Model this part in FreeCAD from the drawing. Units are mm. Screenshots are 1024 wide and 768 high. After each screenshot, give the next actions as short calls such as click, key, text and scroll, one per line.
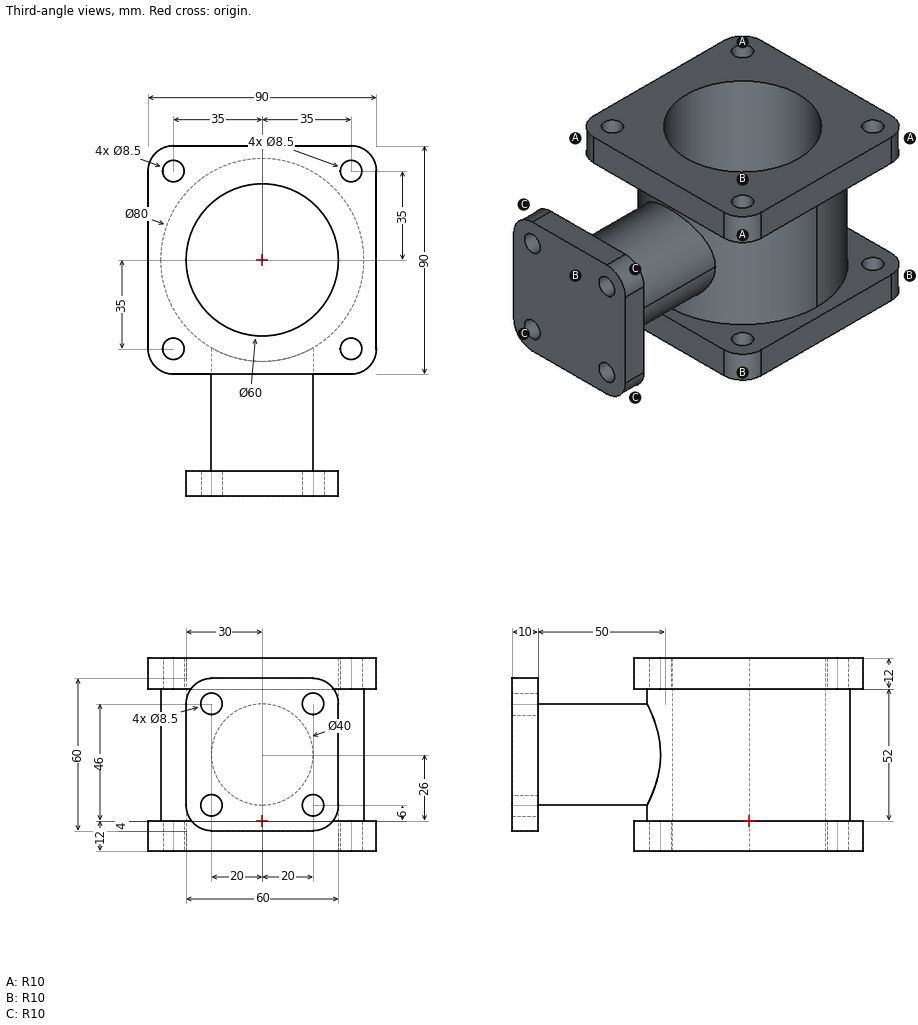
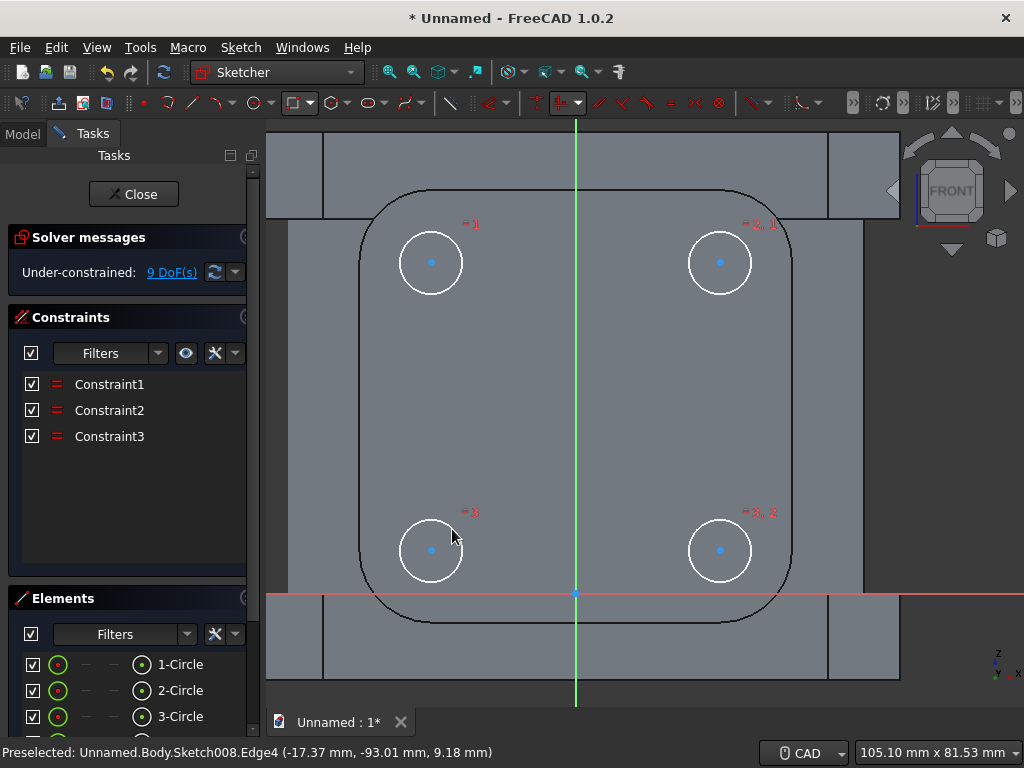
click(431, 263)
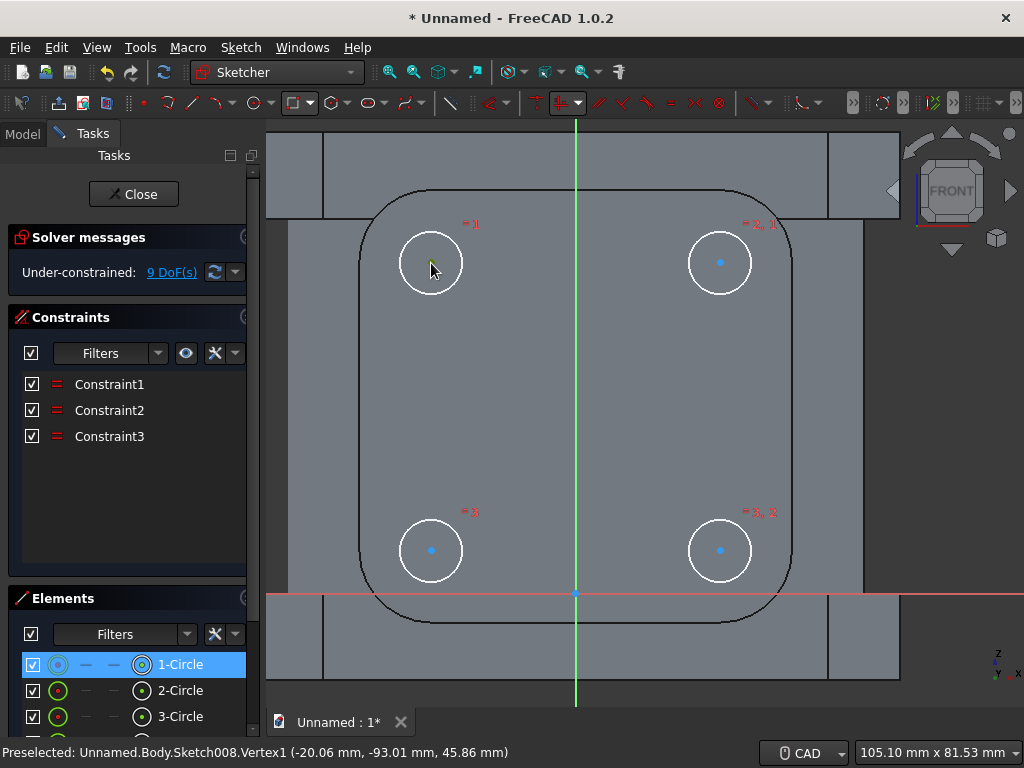
click(720, 263)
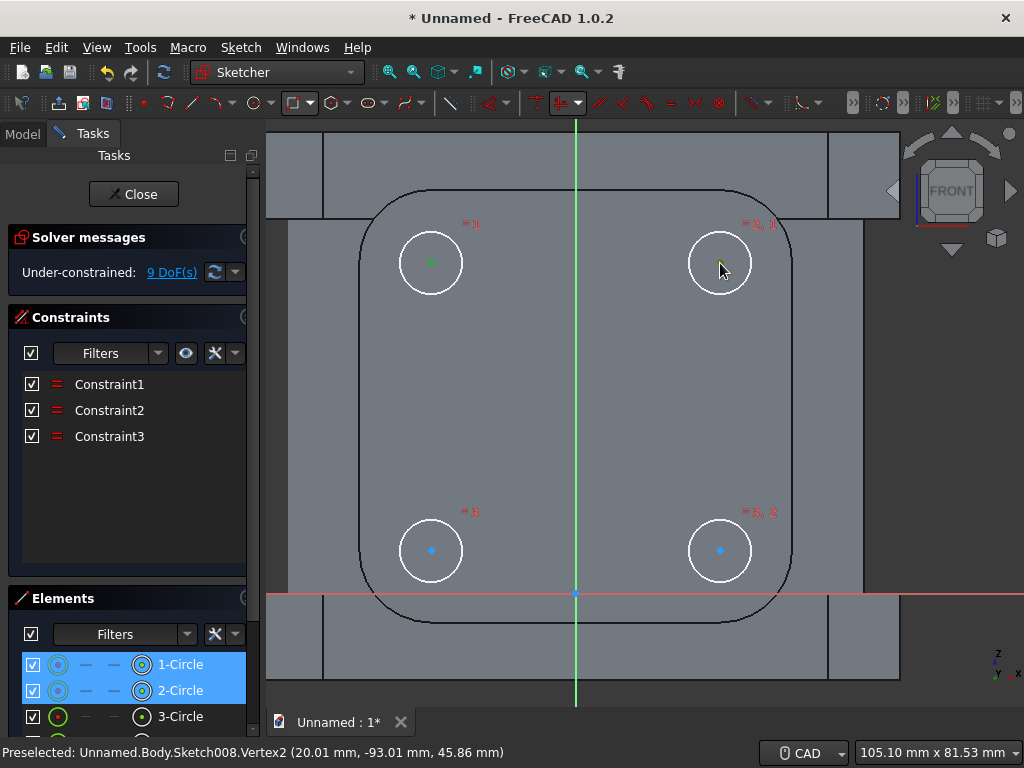
key(h)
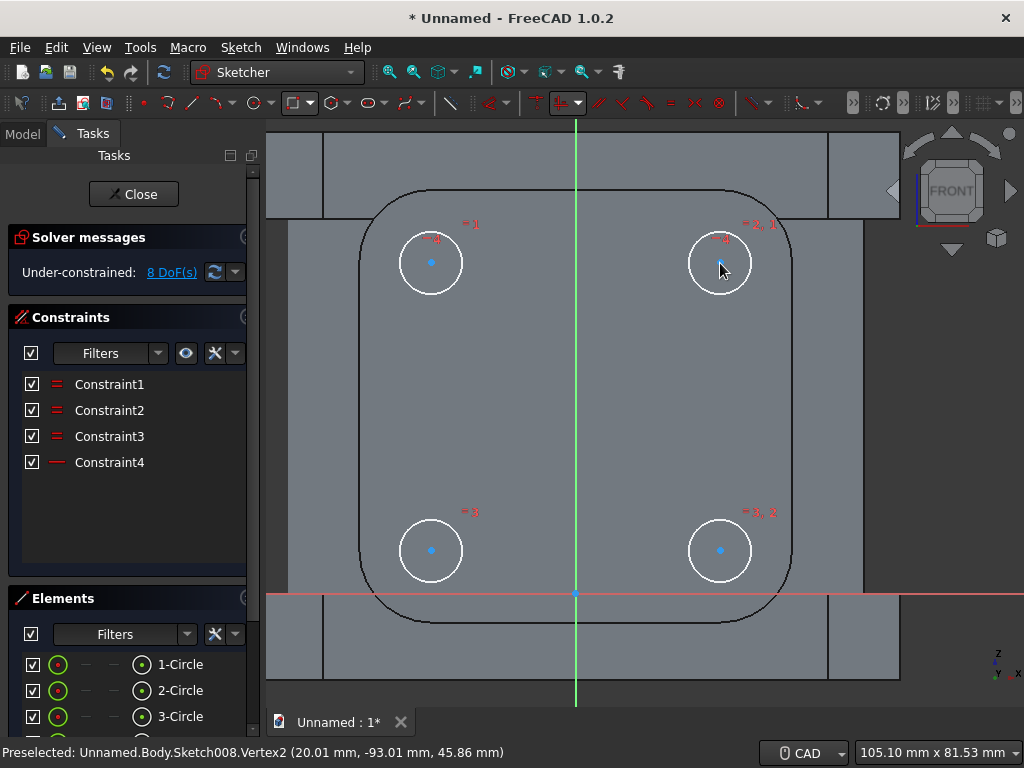
click(720, 263)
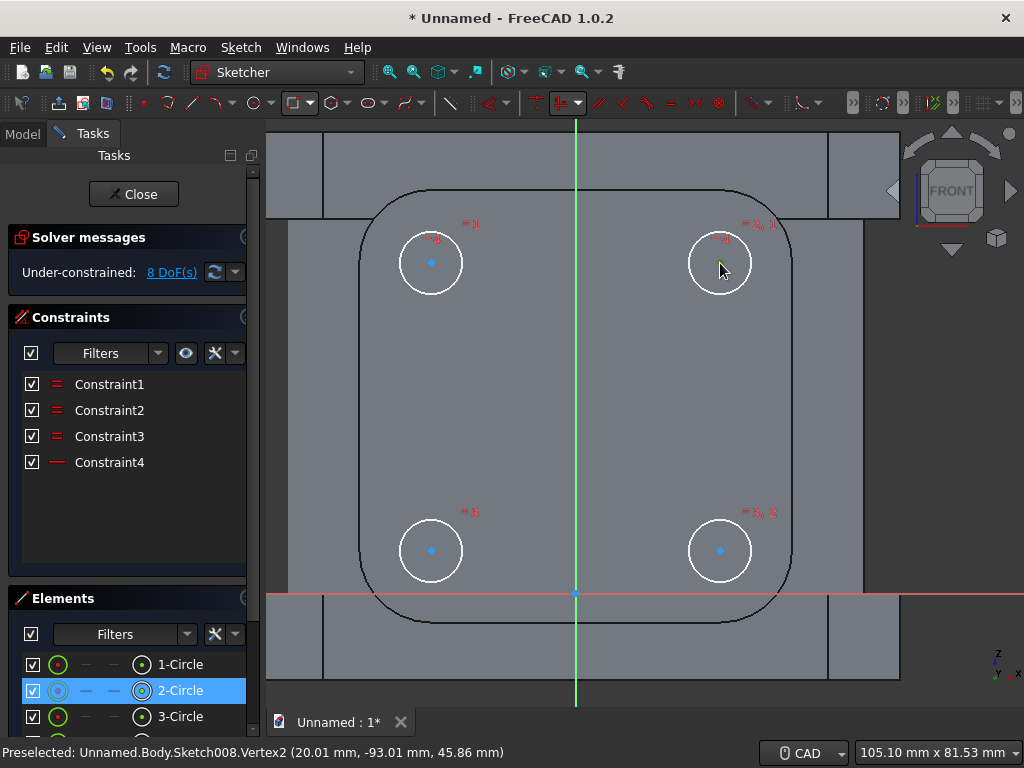
click(720, 551)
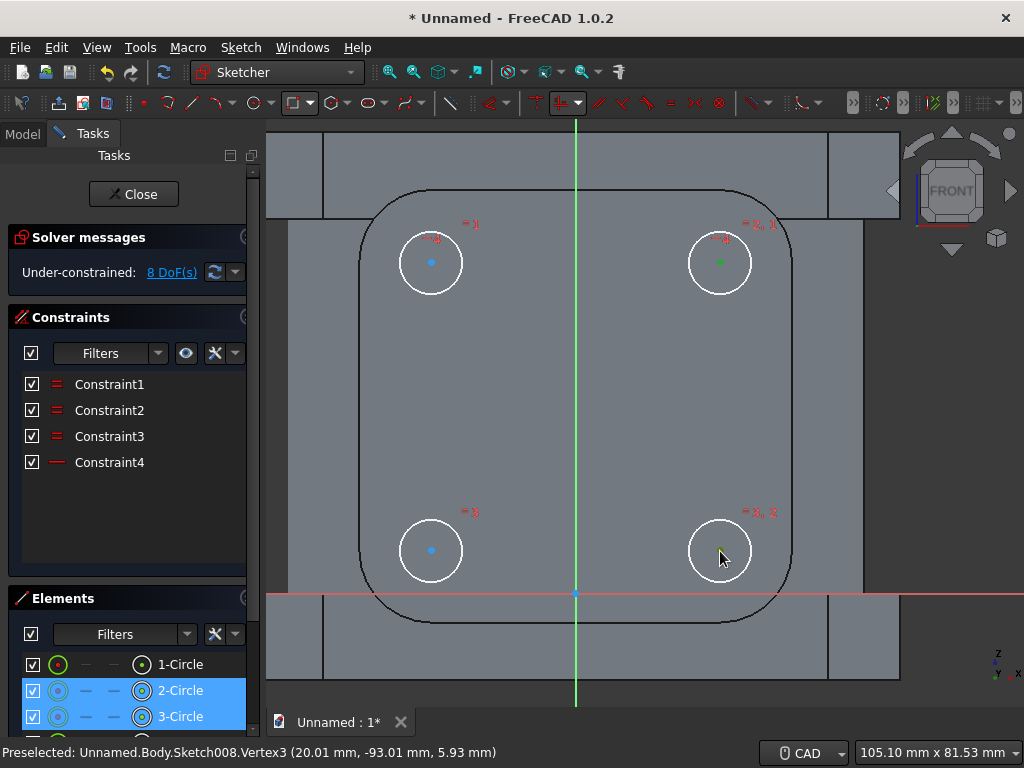
click(580, 104)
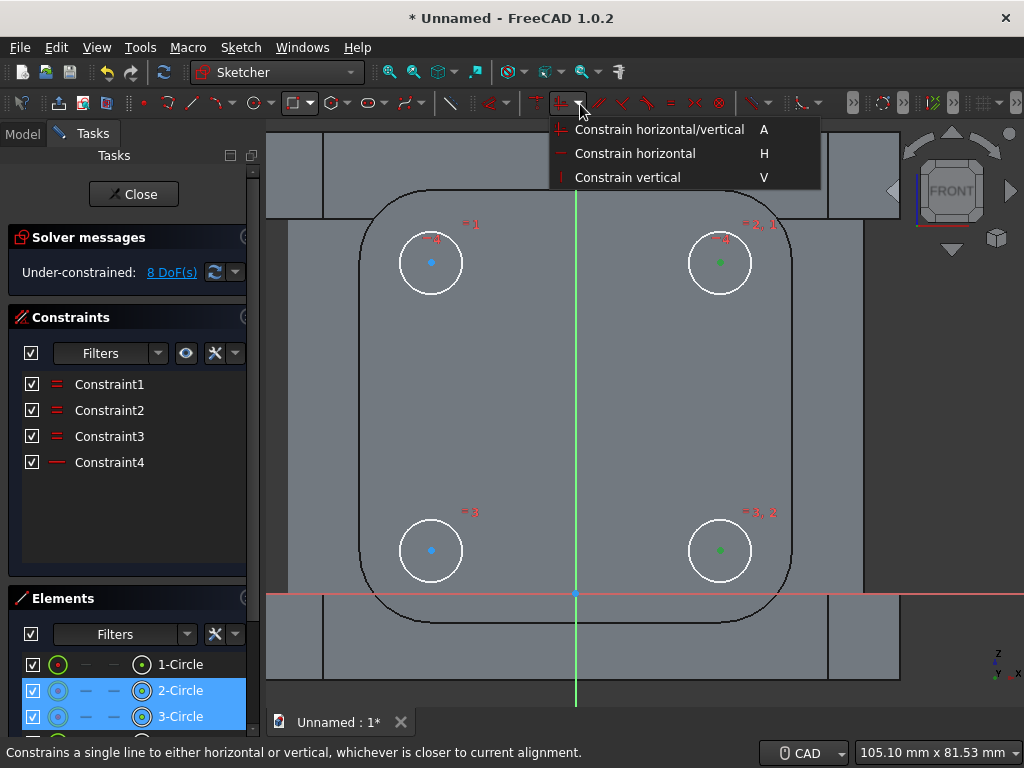
click(685, 177)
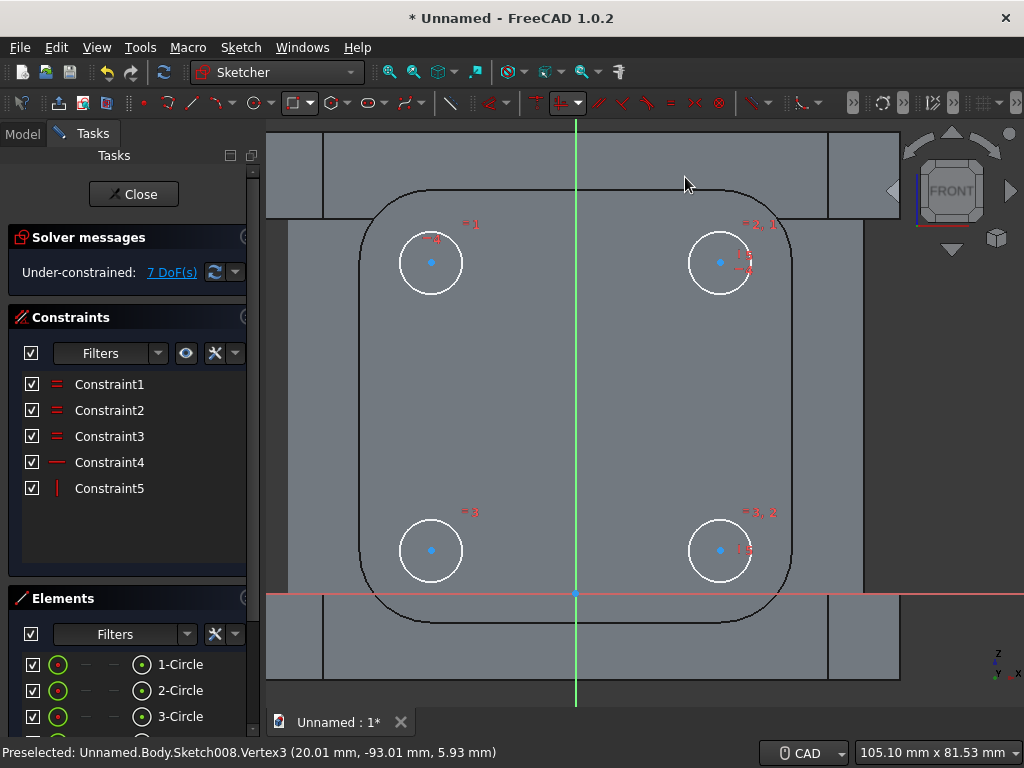
click(431, 263)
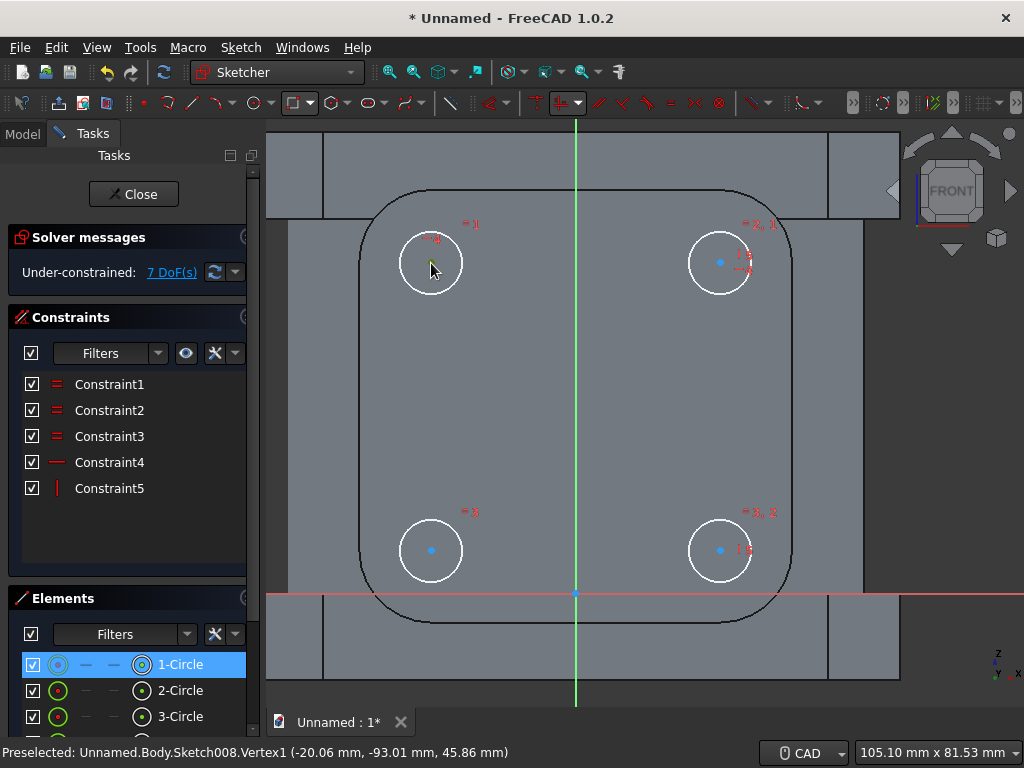
click(431, 551)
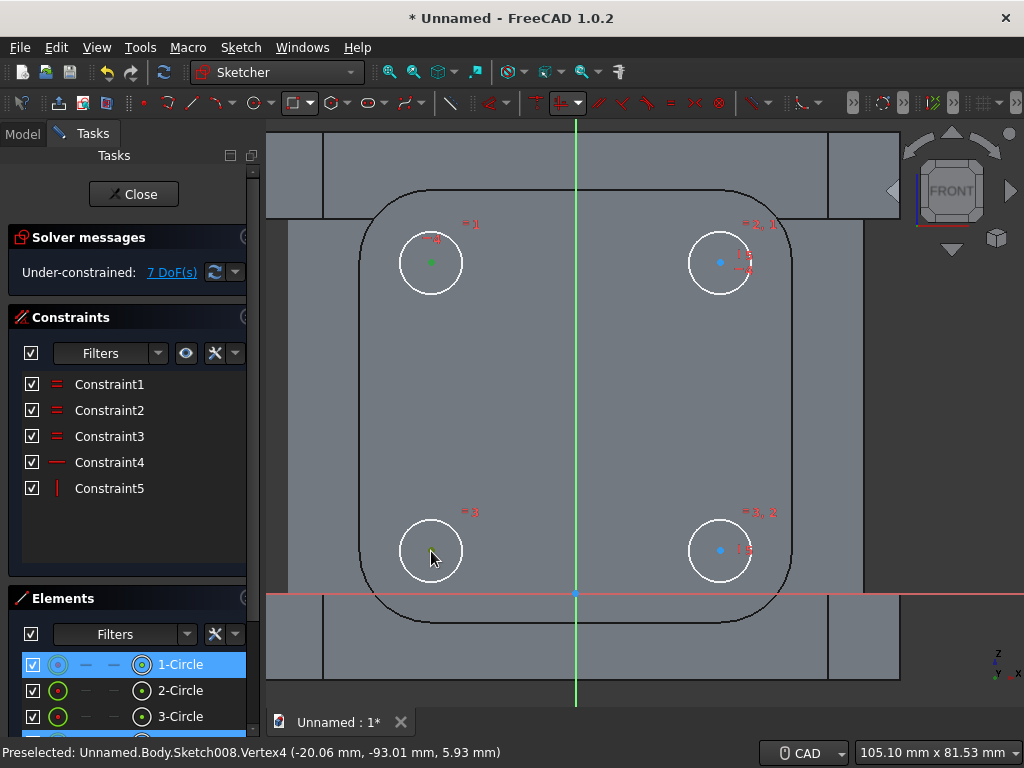
click(580, 104)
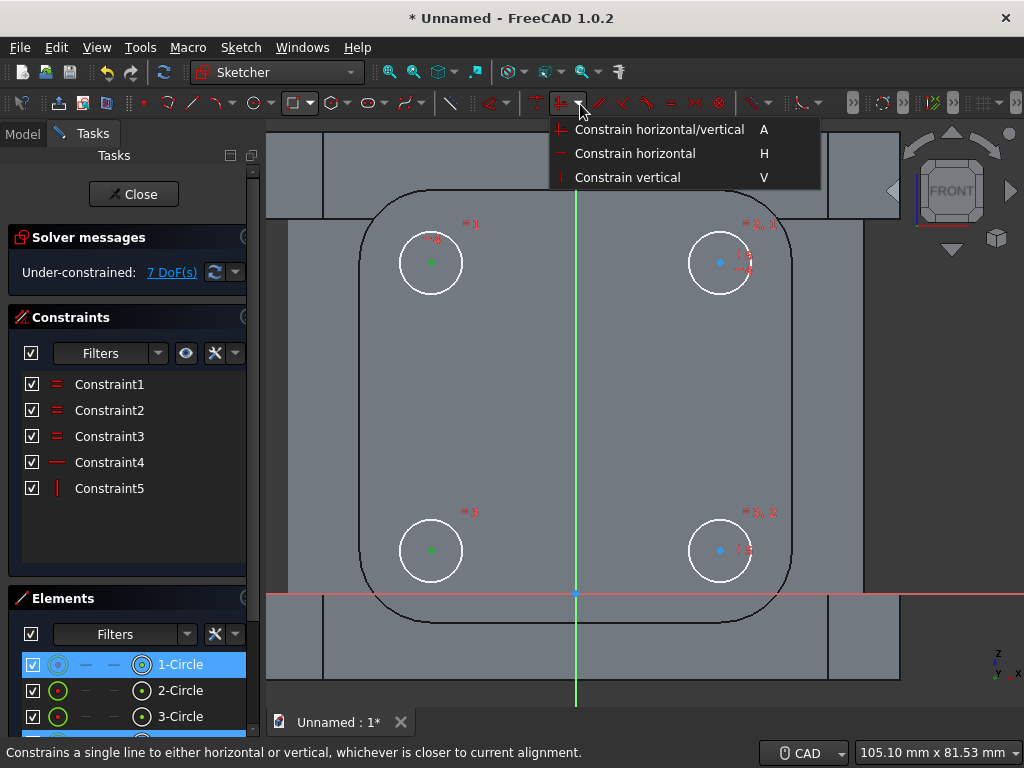
click(685, 177)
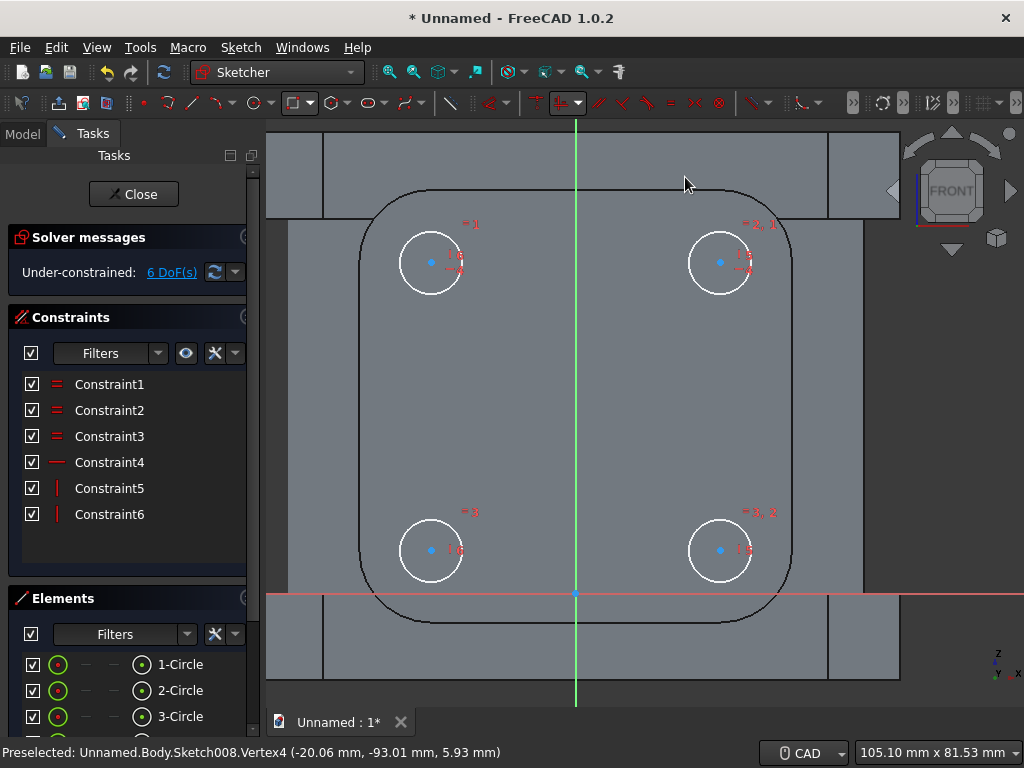
click(720, 551)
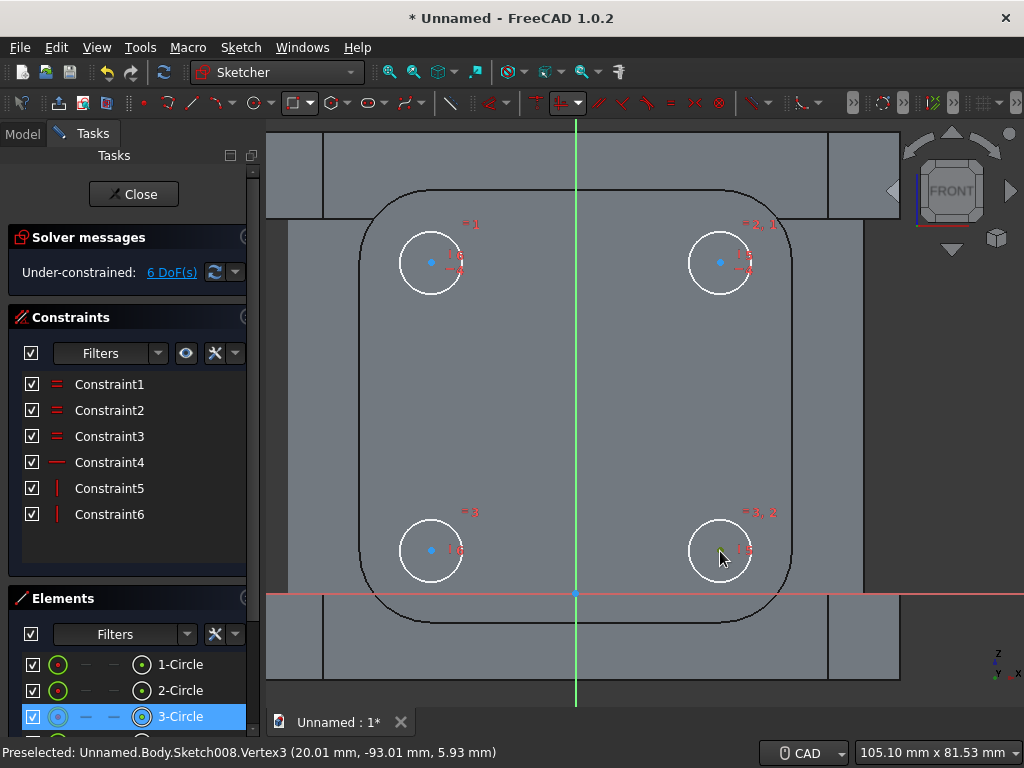
click(431, 551)